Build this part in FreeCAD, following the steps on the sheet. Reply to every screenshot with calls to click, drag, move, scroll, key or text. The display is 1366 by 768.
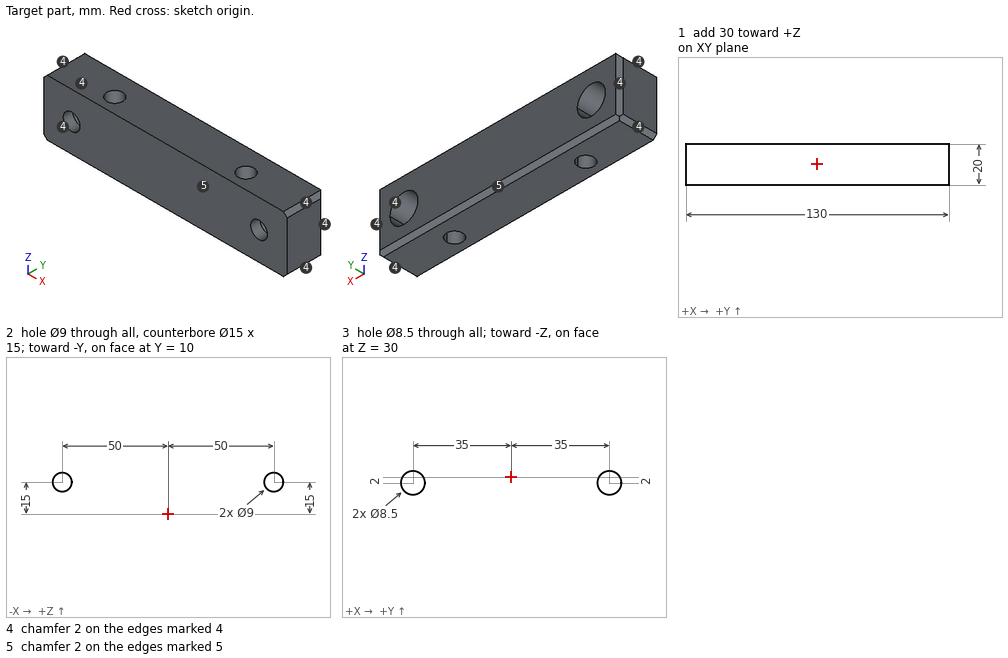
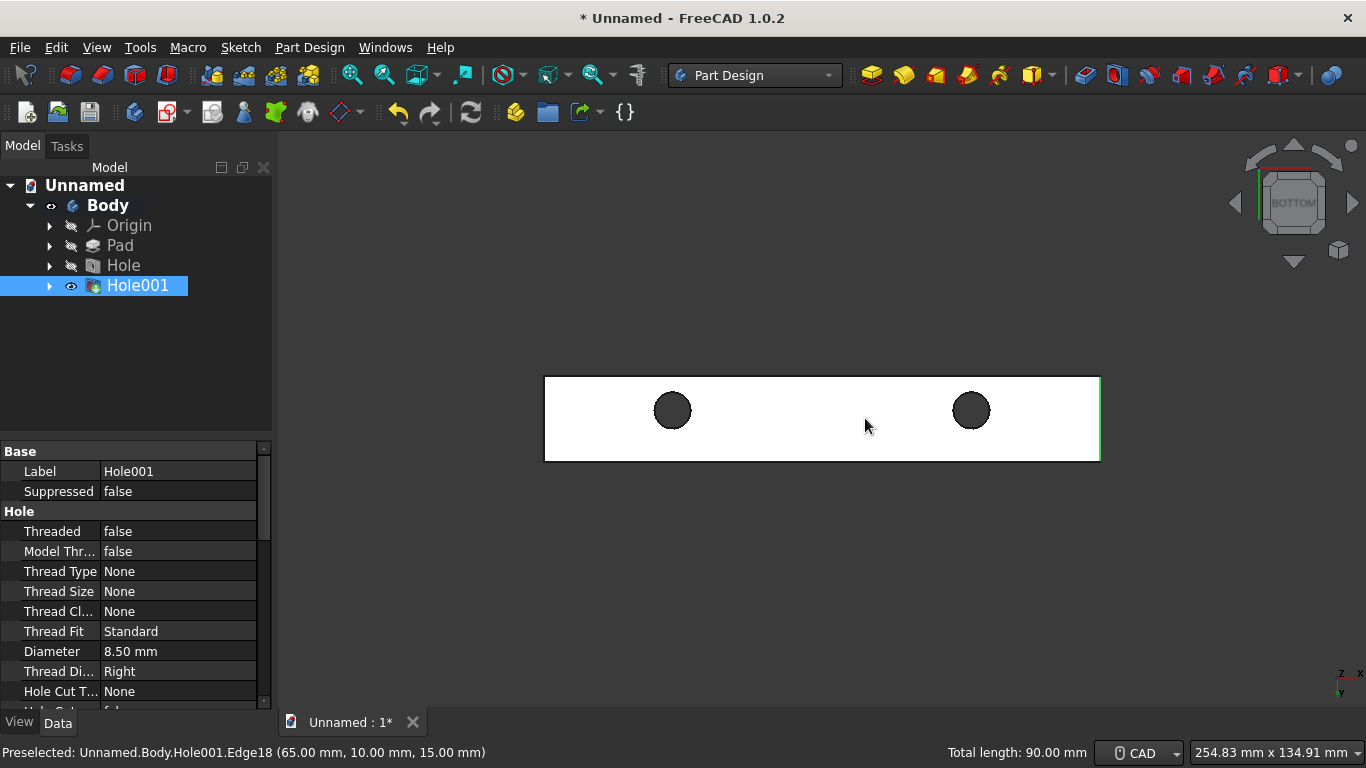
click(544, 418, ctrl)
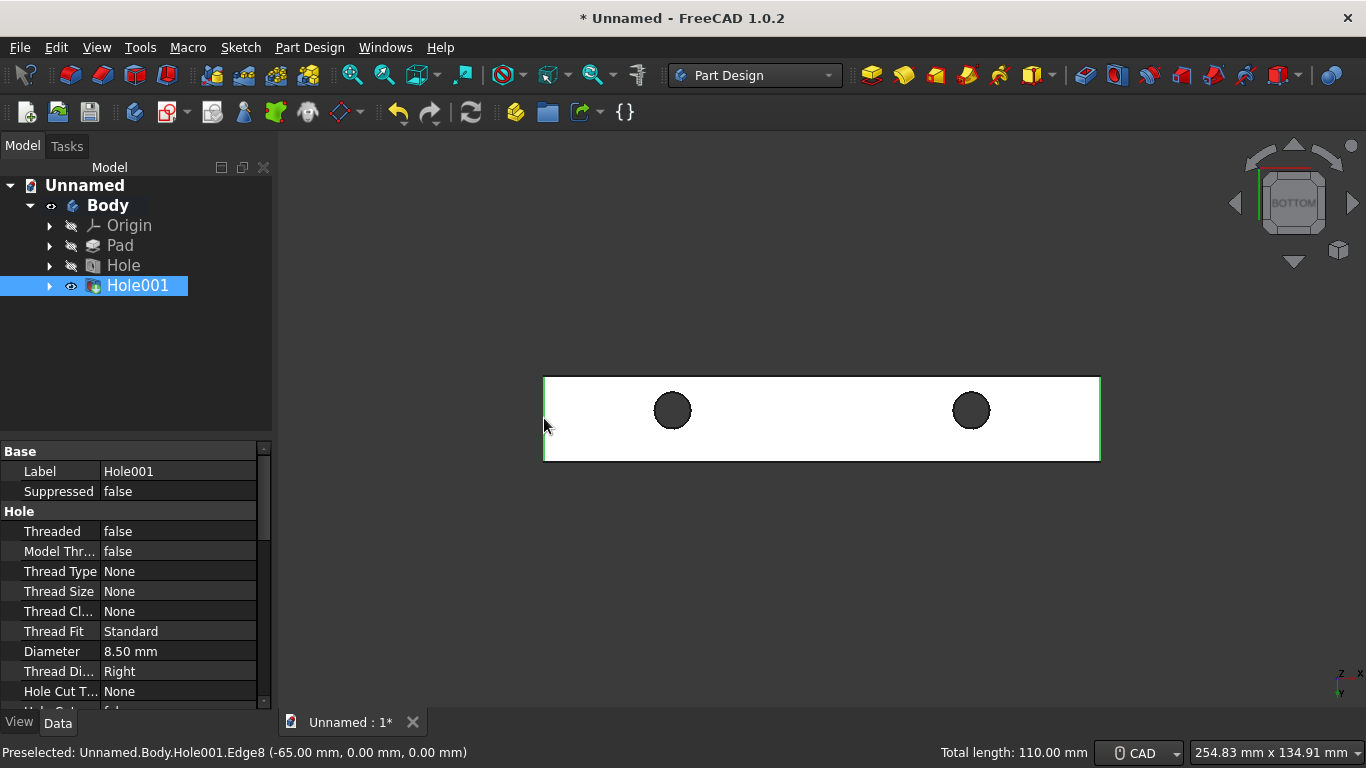
key(4)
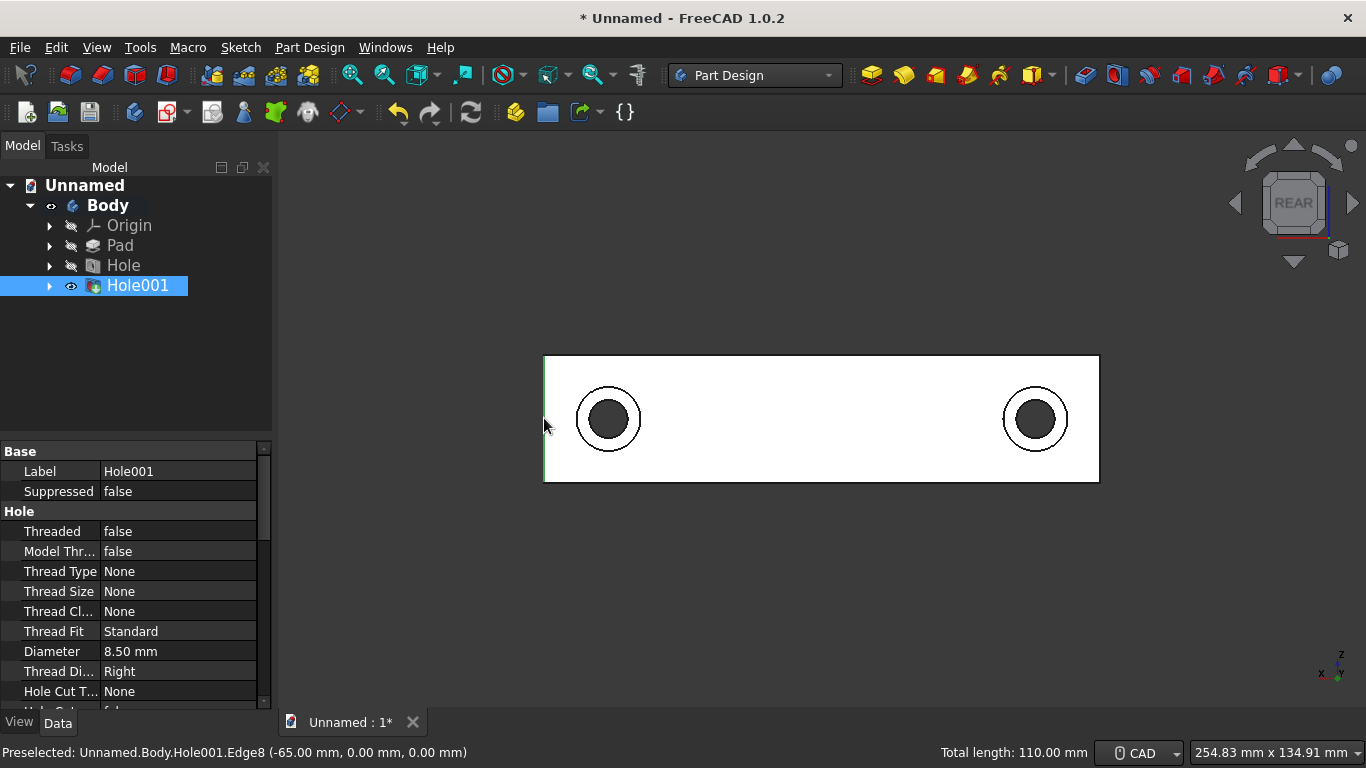
click(1100, 418, ctrl)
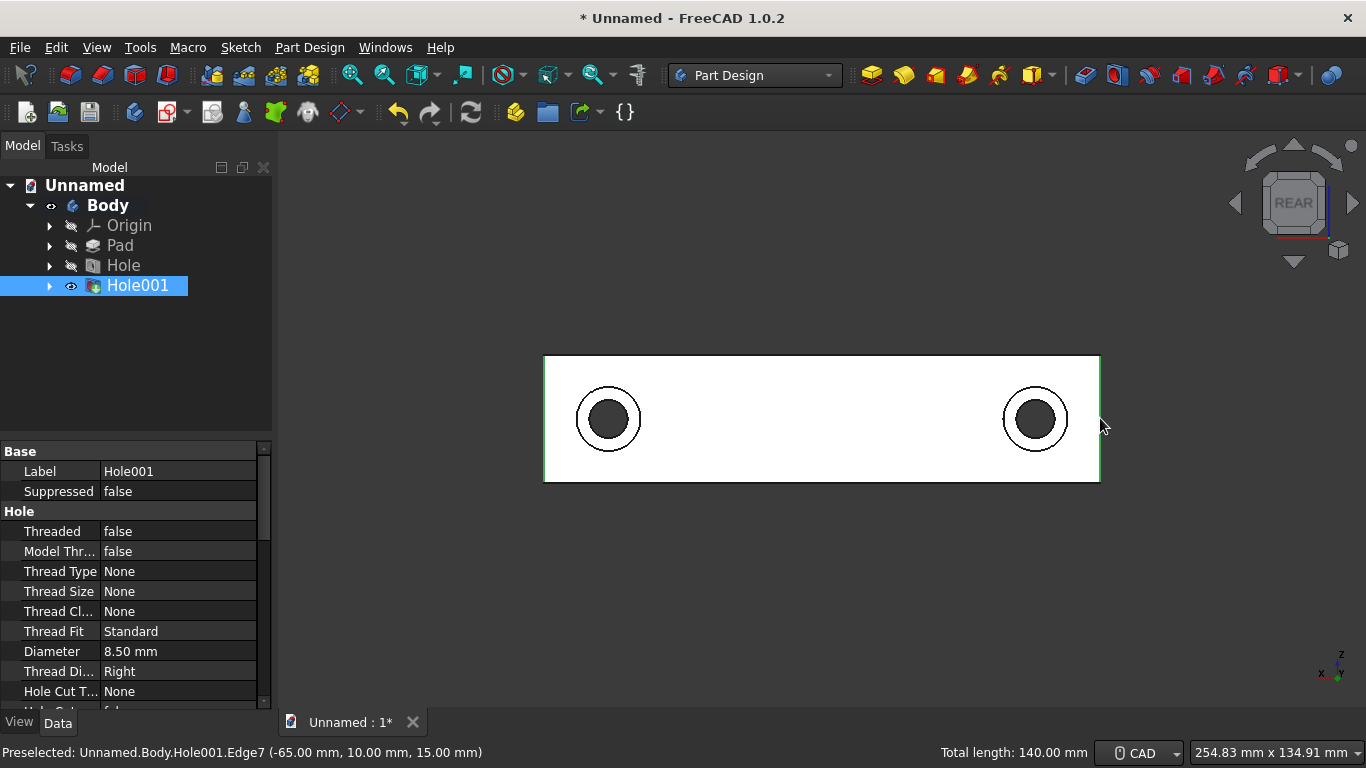
click(104, 76)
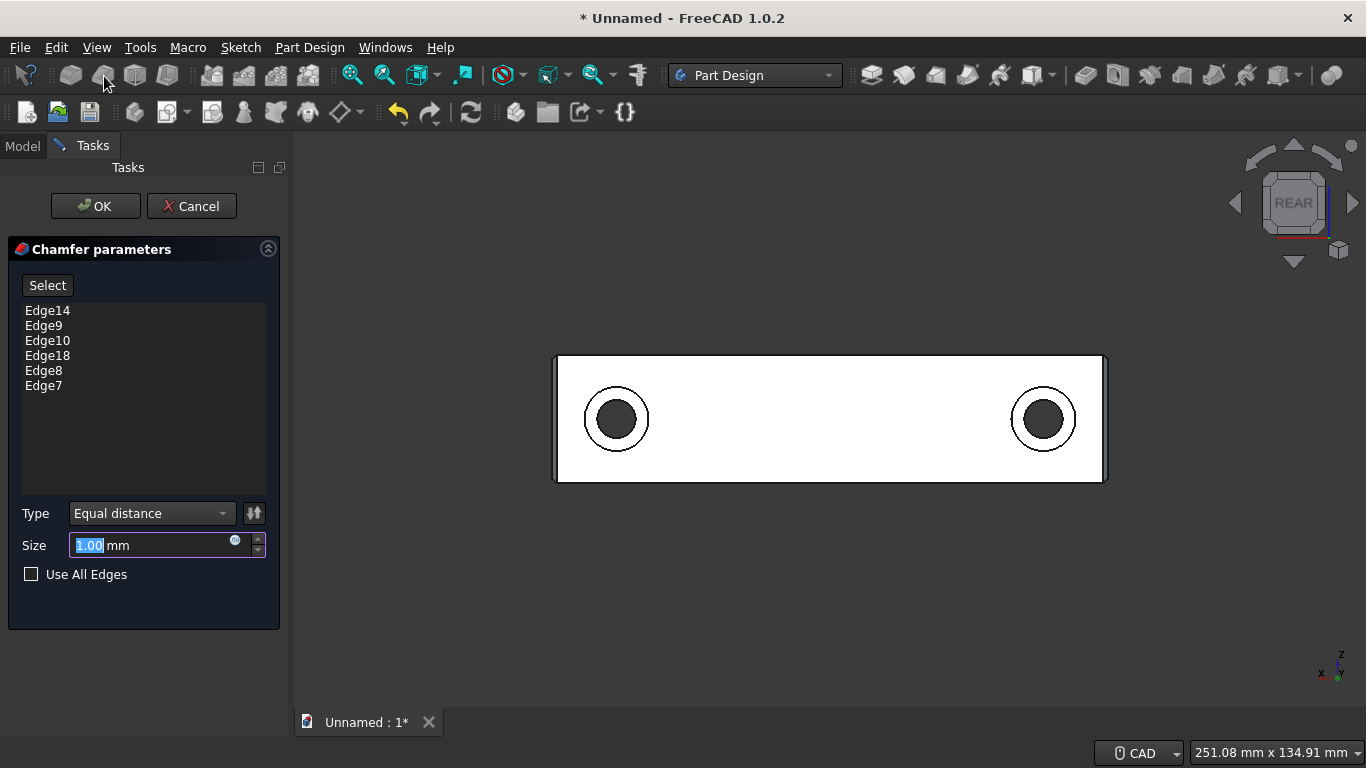
text(2)
key(Tab)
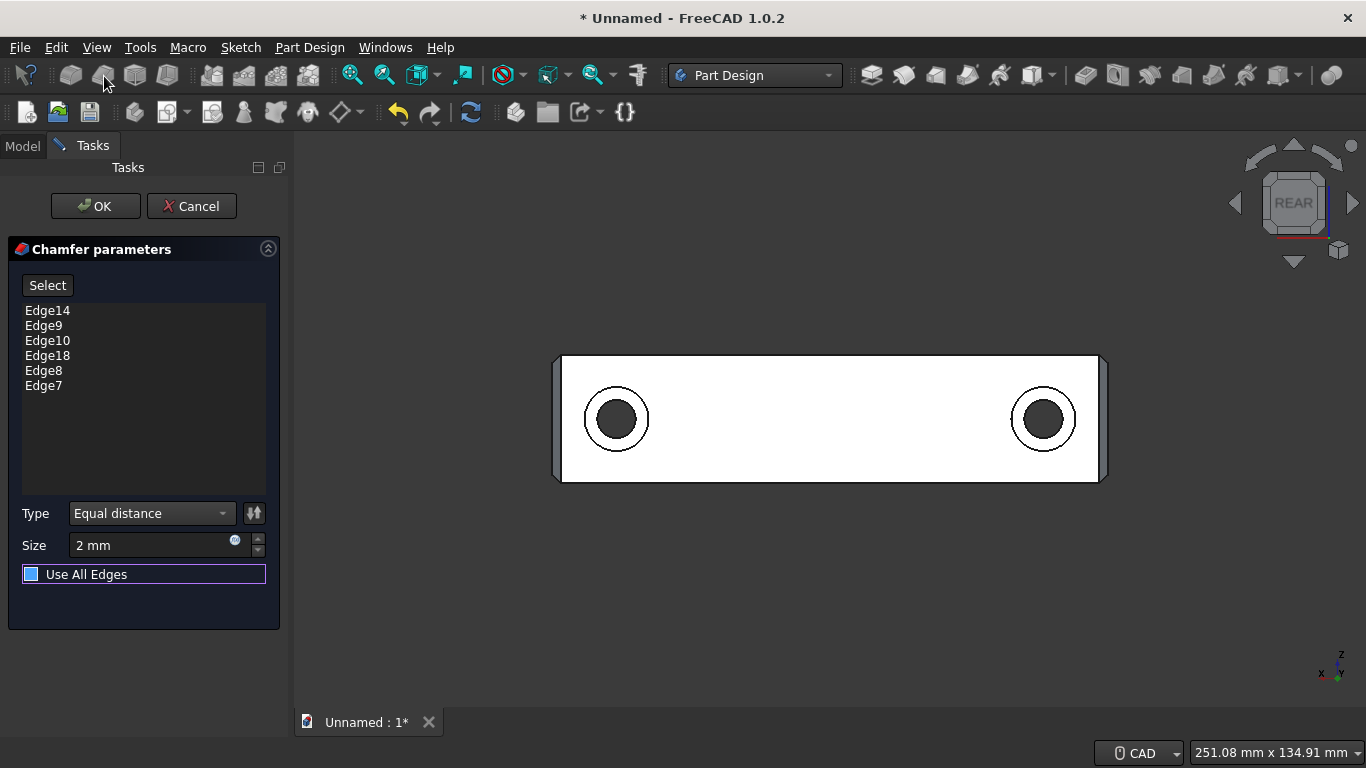
click(96, 206)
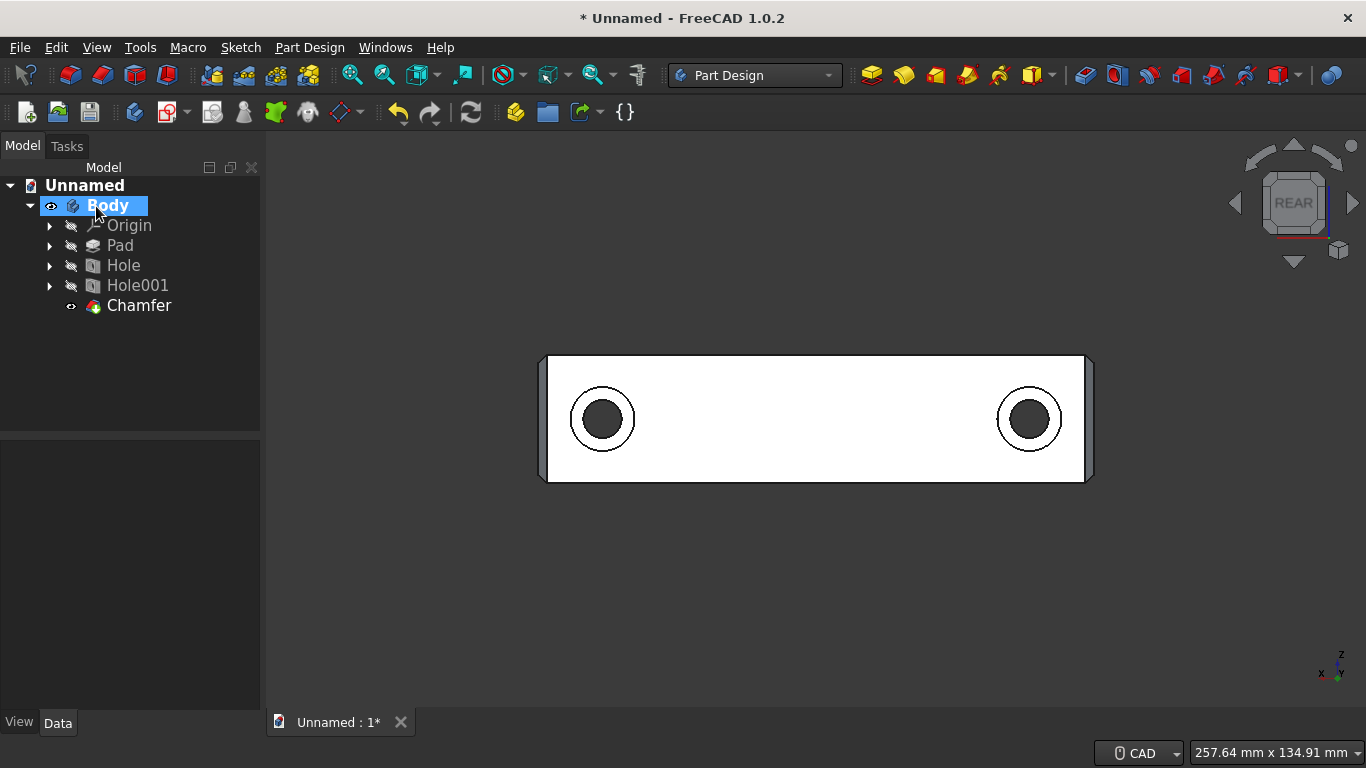
click(816, 482)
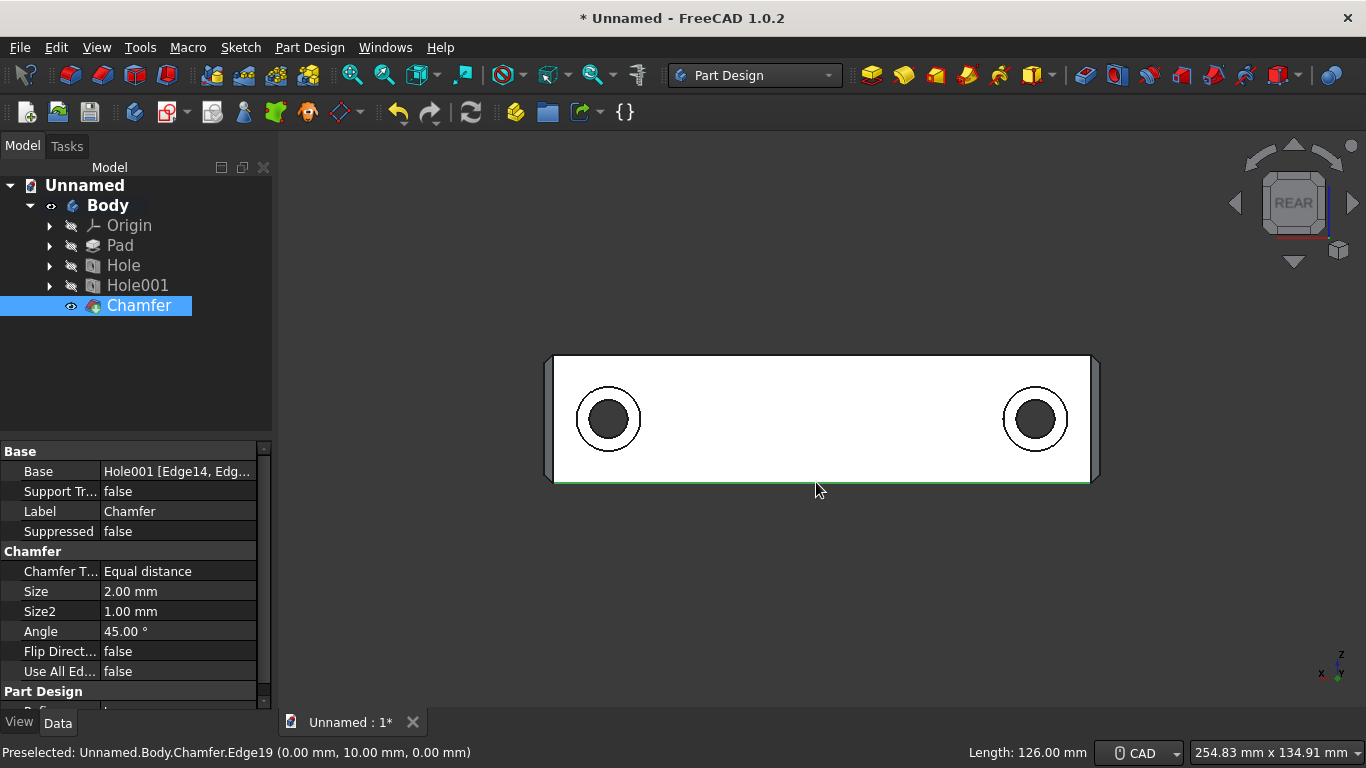
click(104, 76)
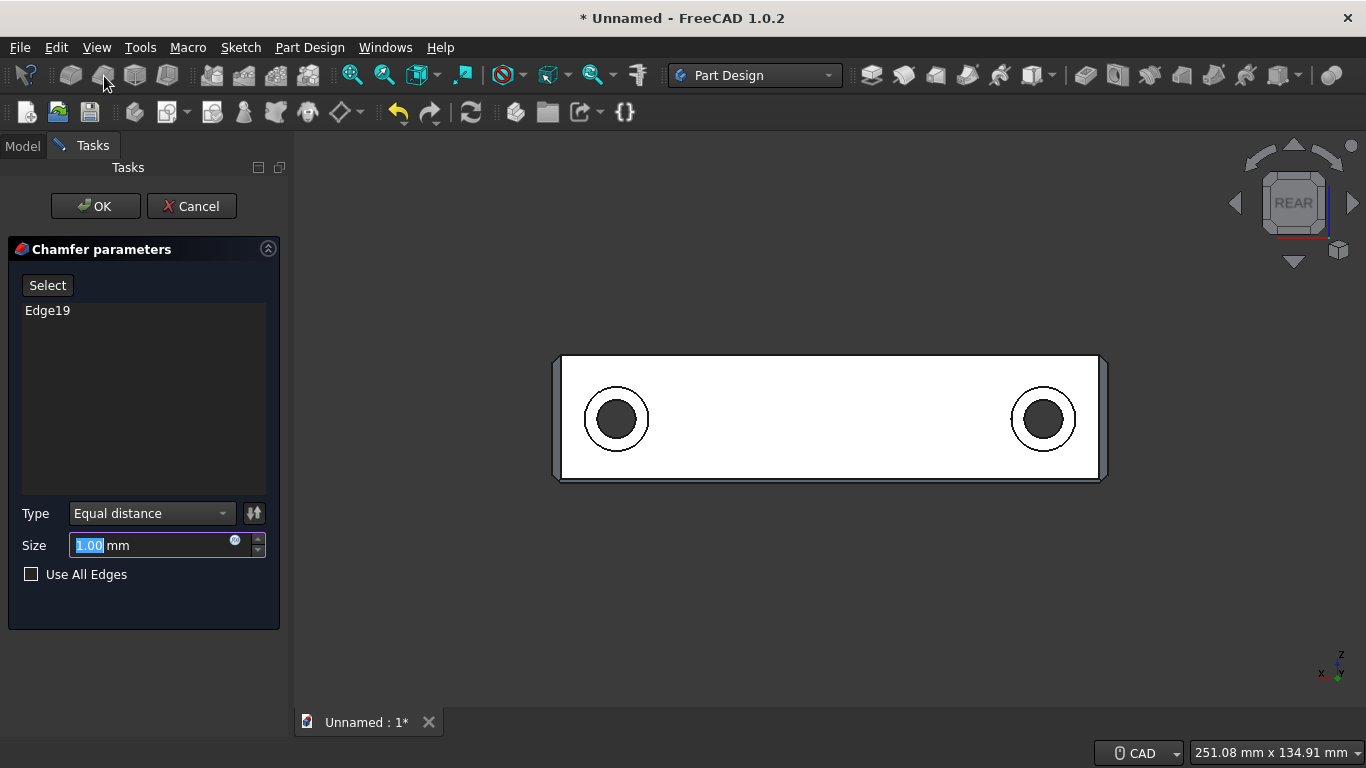
text(2)
key(Tab)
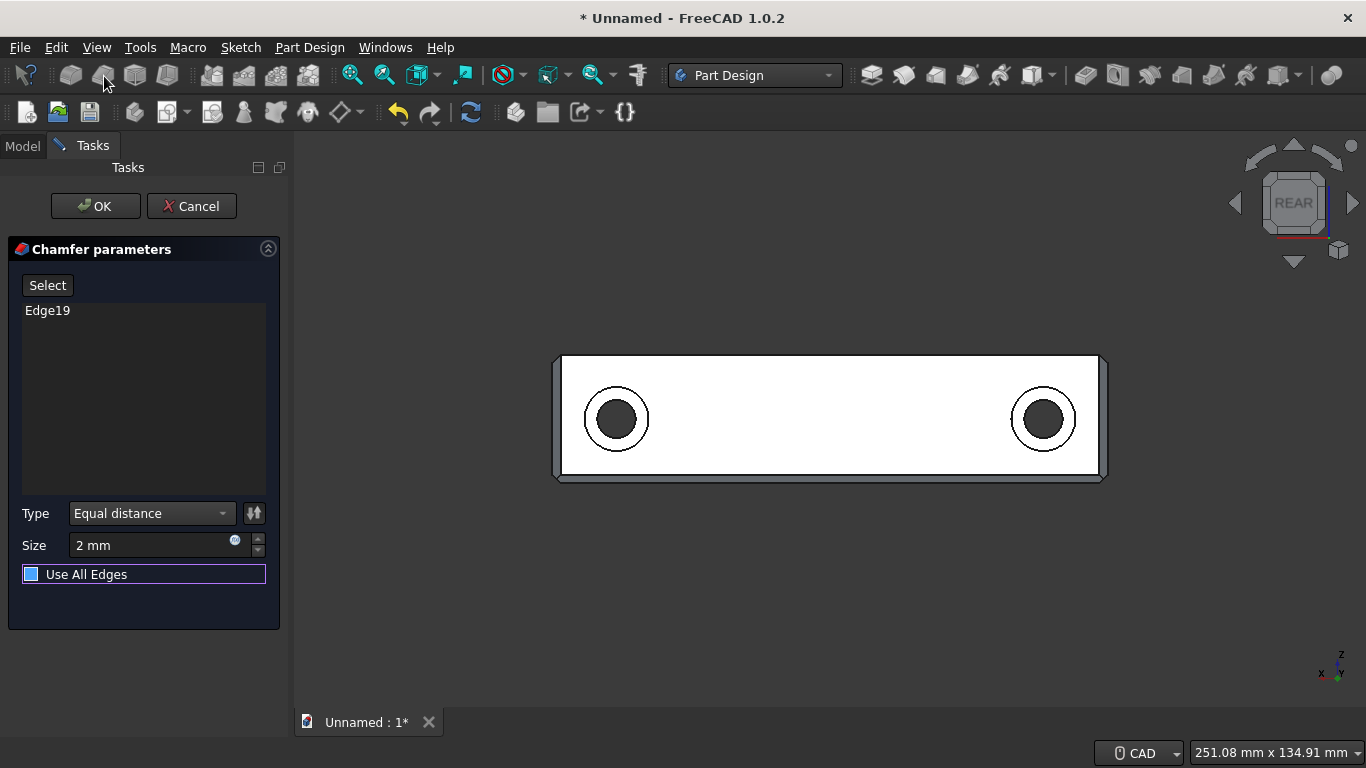
click(96, 206)